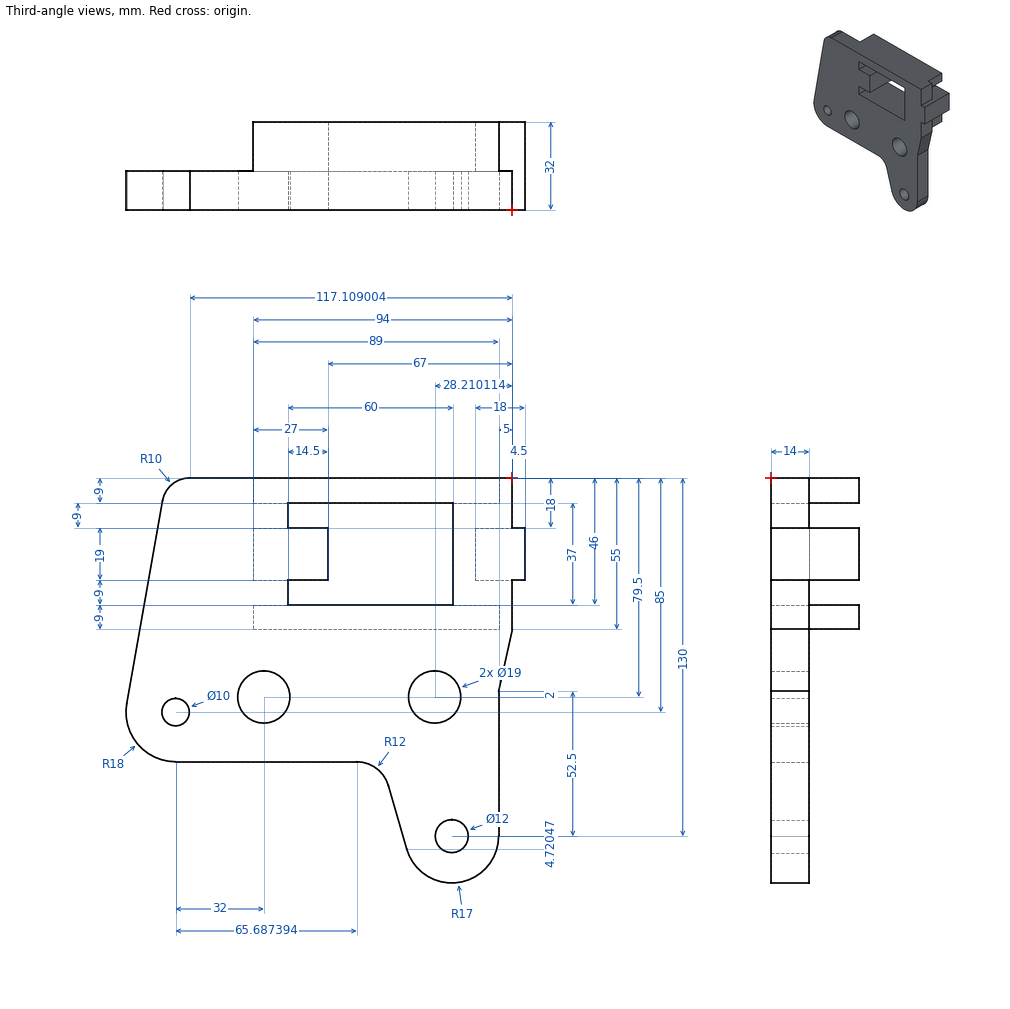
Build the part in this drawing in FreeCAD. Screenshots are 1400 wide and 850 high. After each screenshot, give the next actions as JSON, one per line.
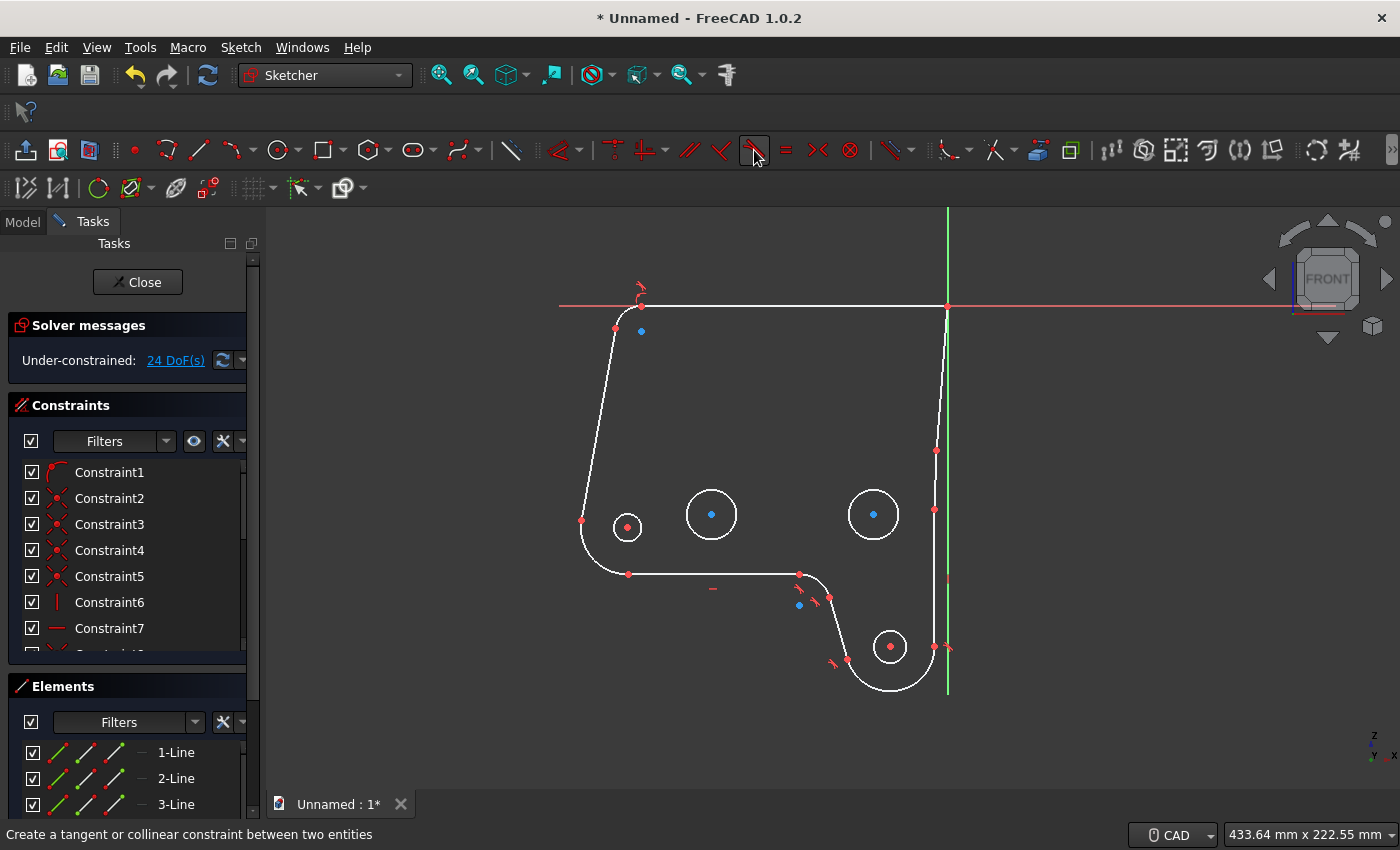
{"action": "left_click", "coordinate": [748, 574]}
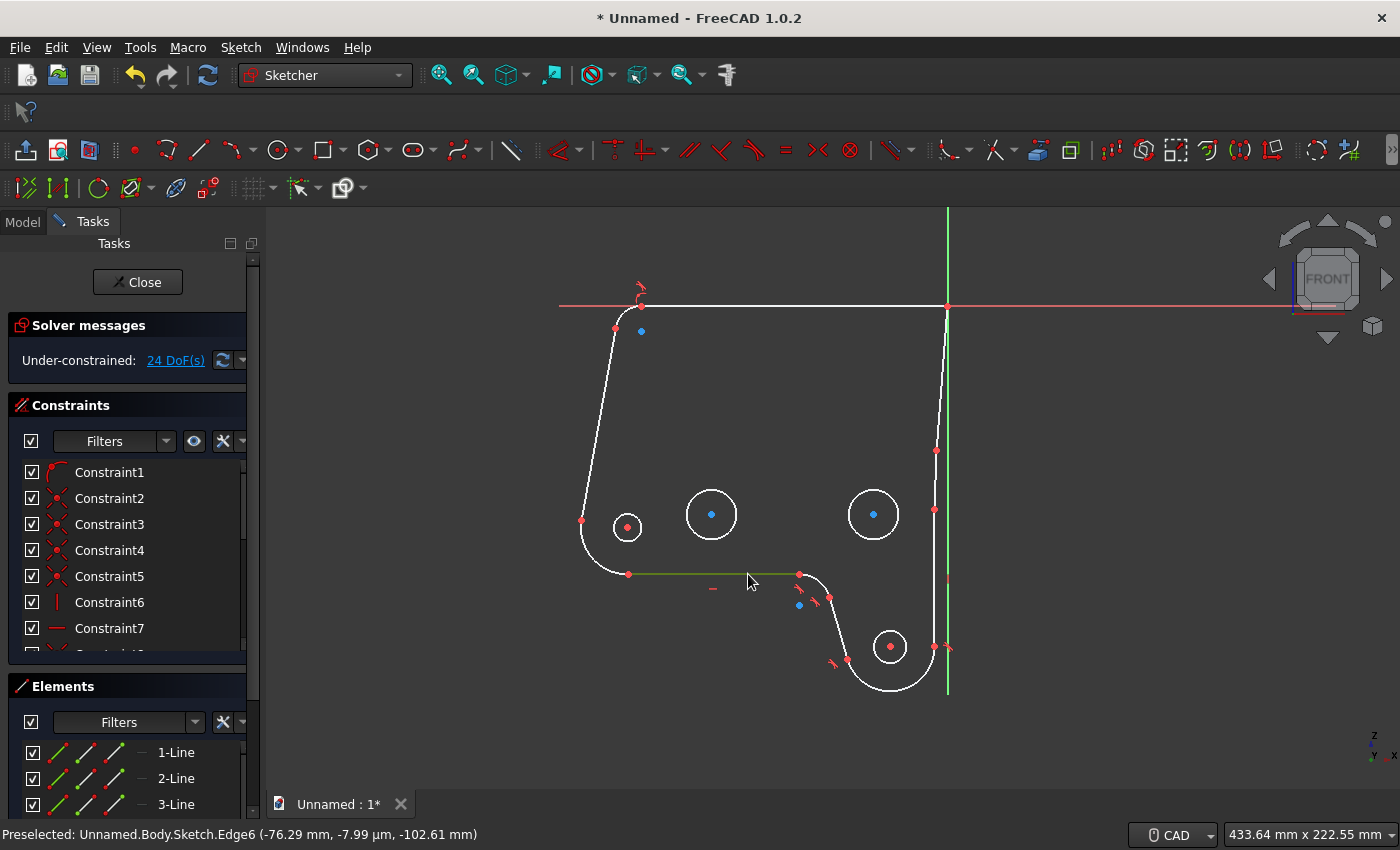
{"action": "left_click", "coordinate": [584, 545]}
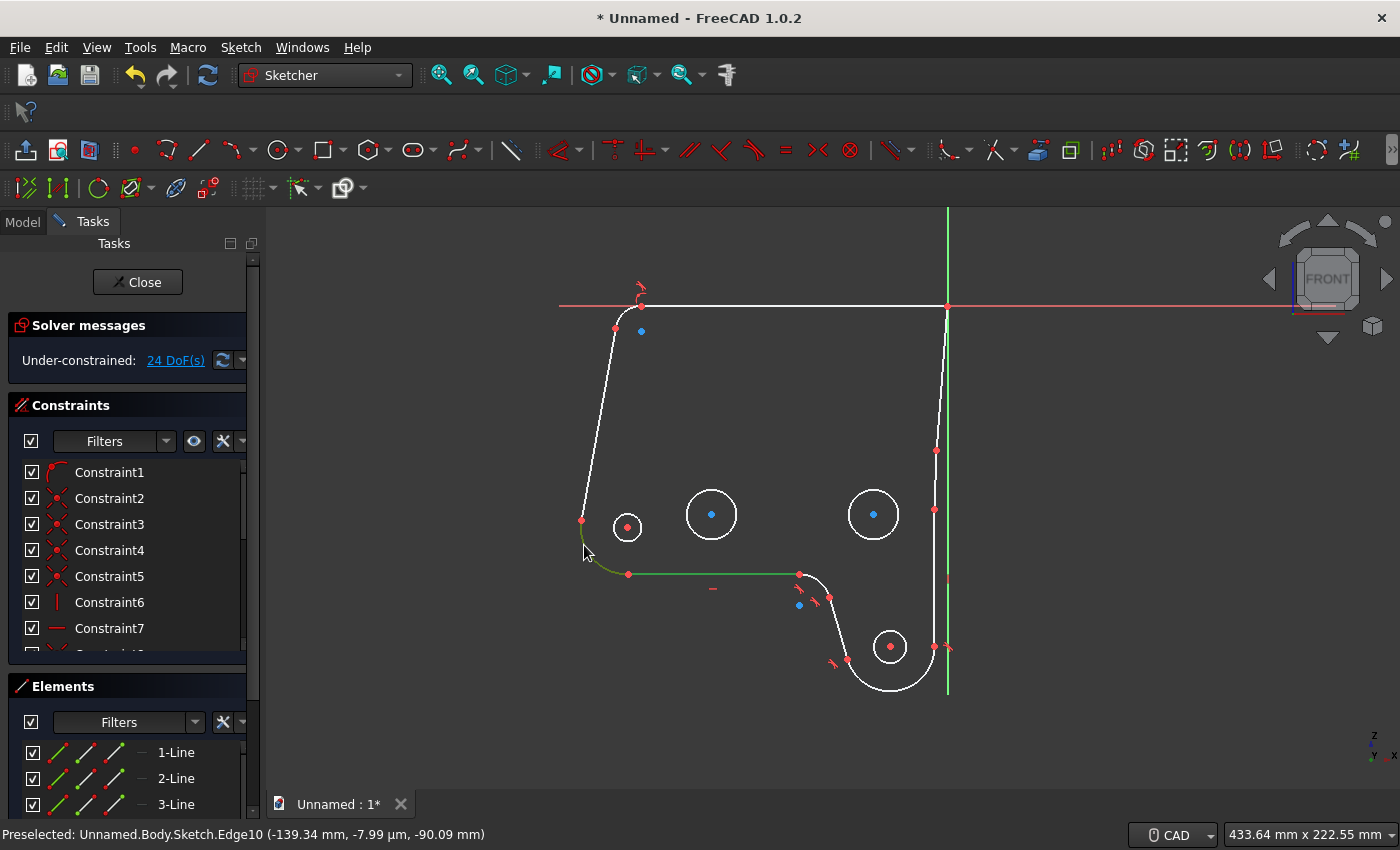
{"action": "left_click", "coordinate": [754, 150]}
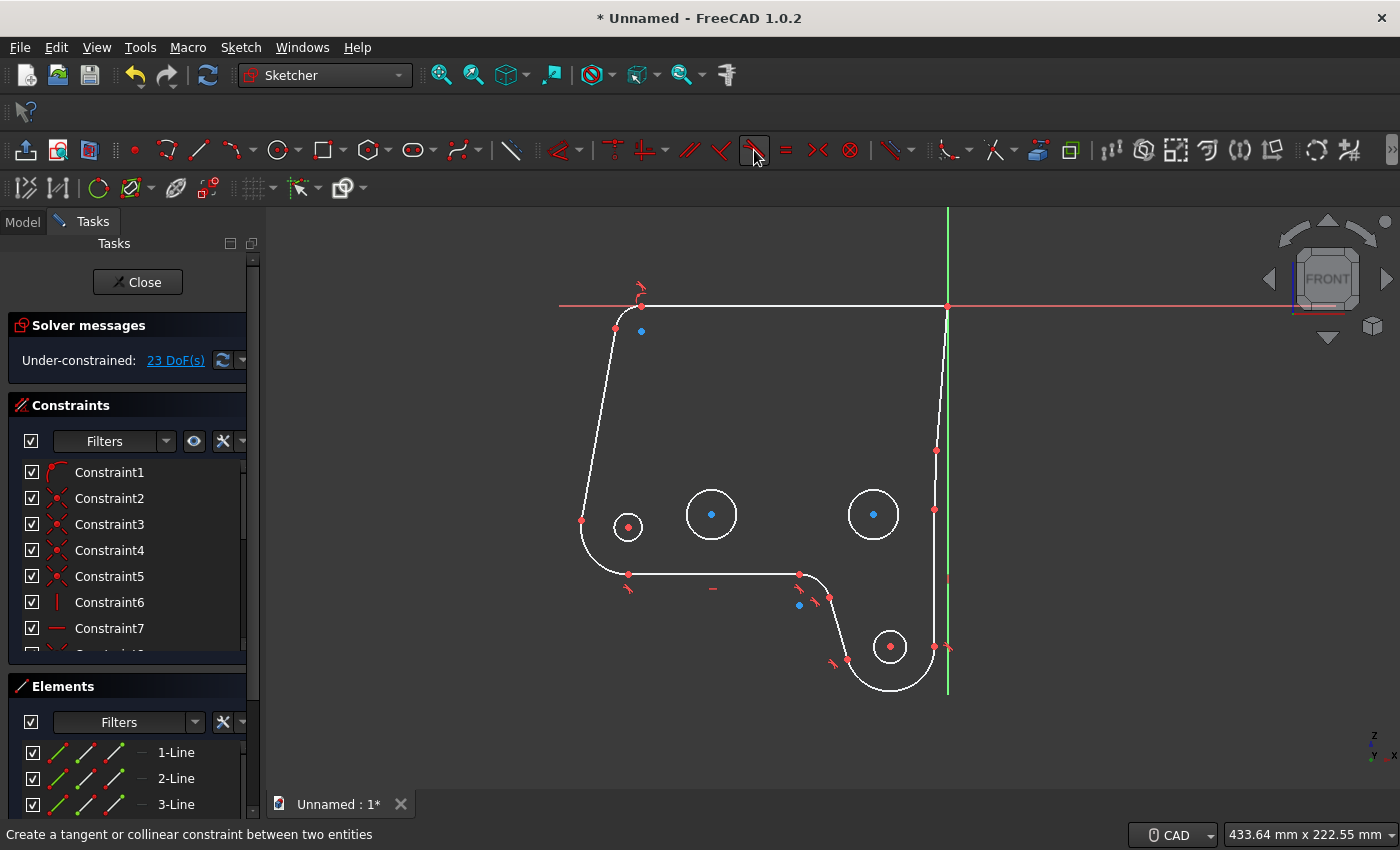
{"action": "left_click", "coordinate": [592, 463]}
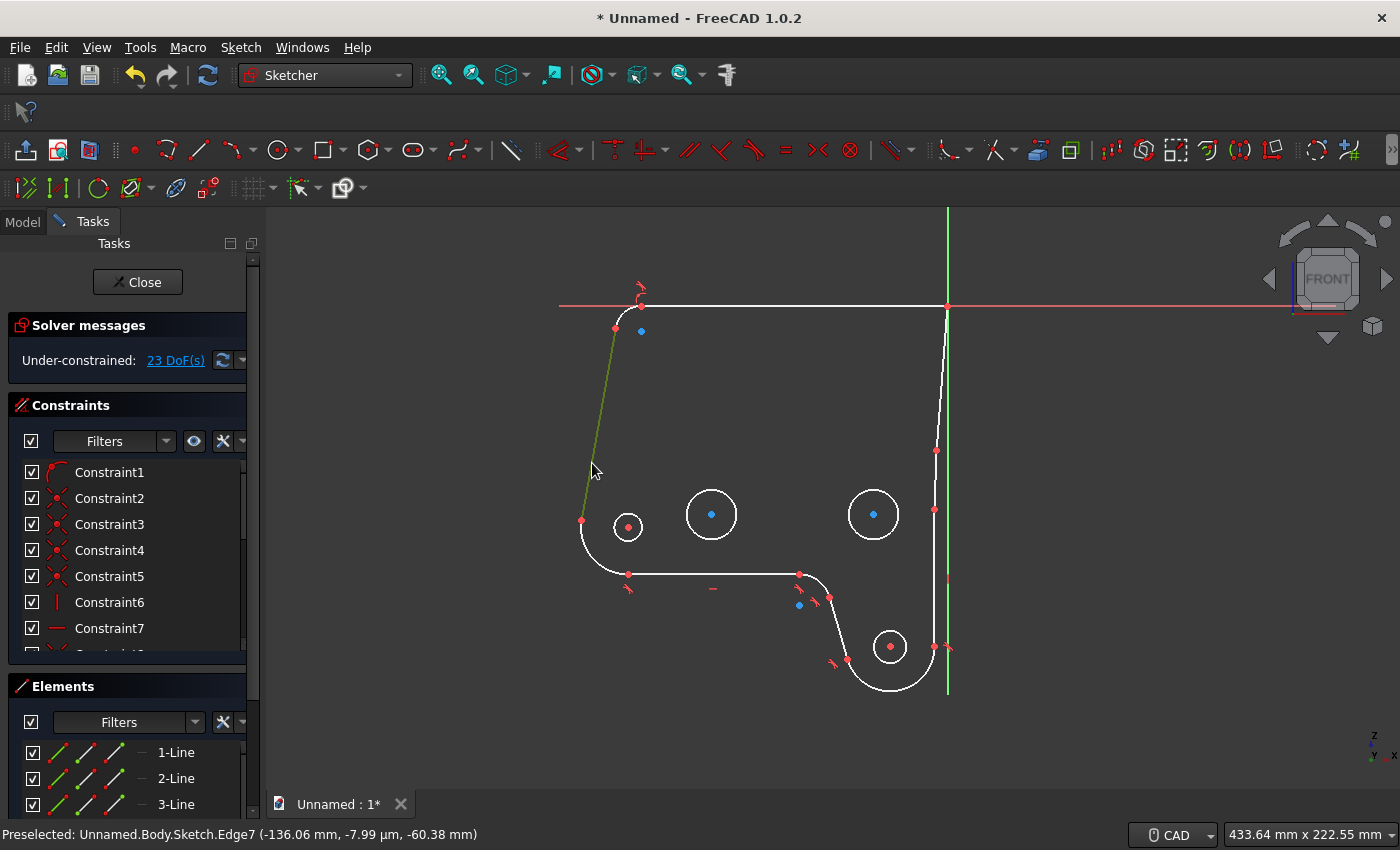
{"action": "left_click", "coordinate": [584, 545]}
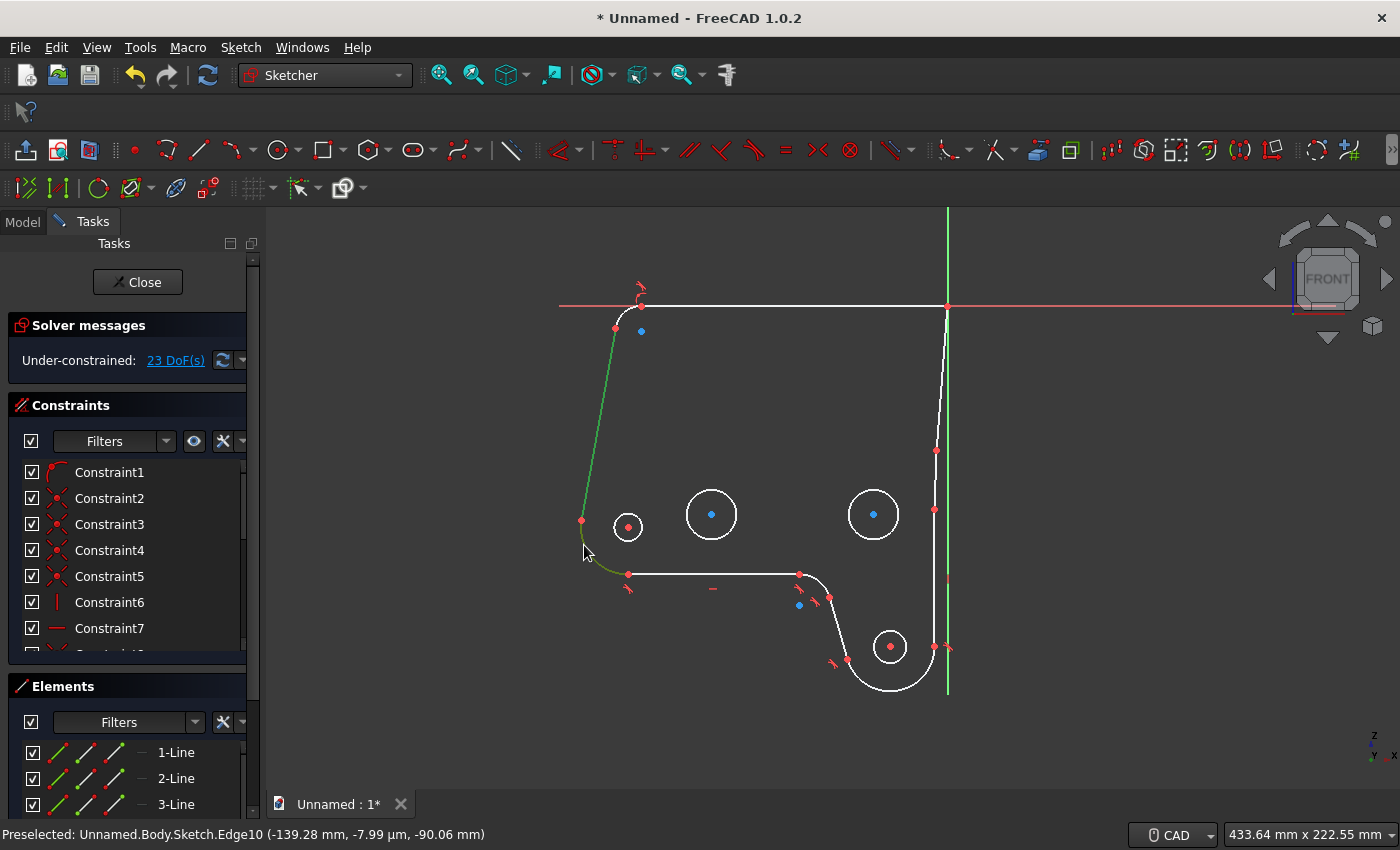
{"action": "left_click", "coordinate": [754, 150]}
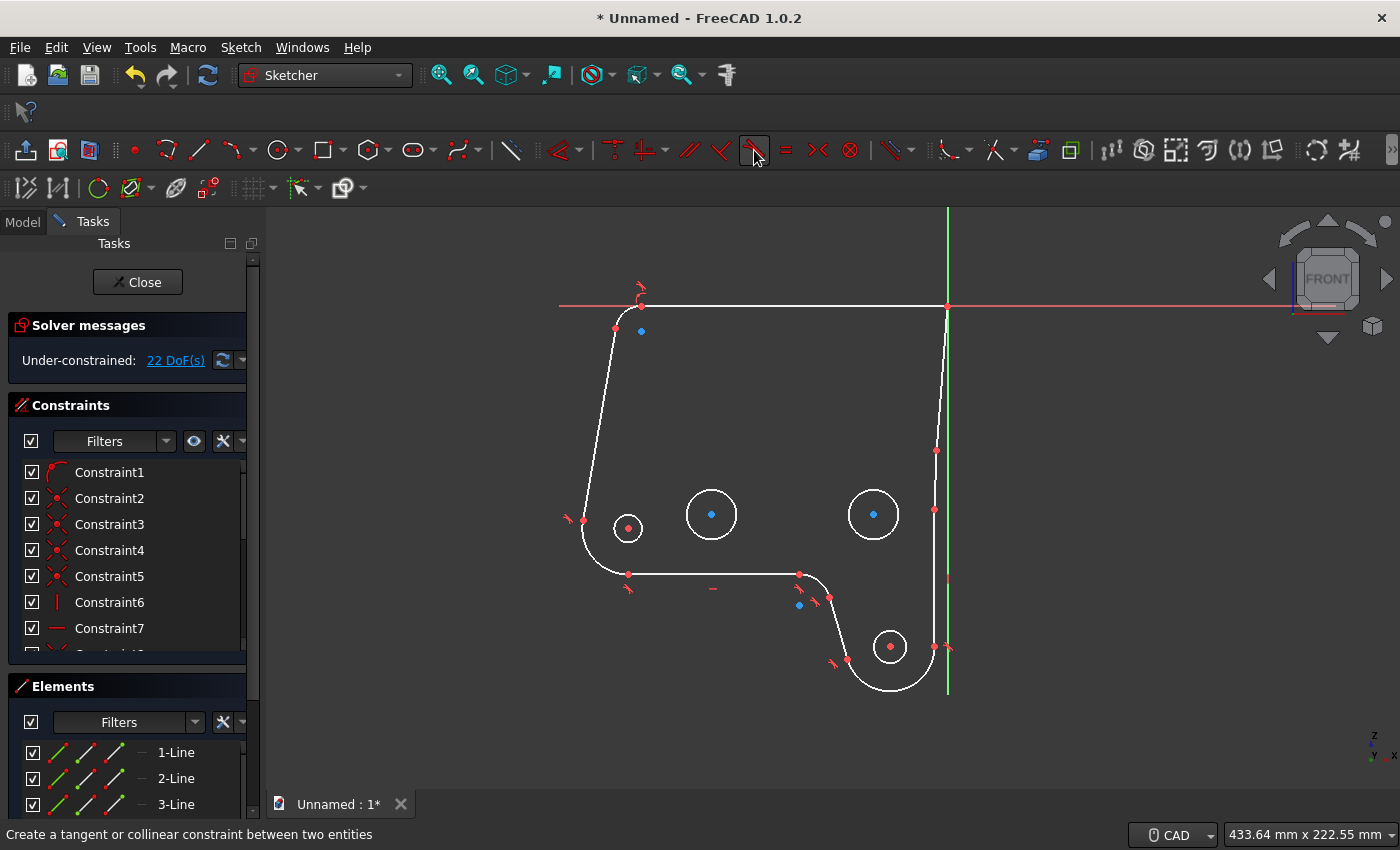
{"action": "left_click", "coordinate": [593, 463]}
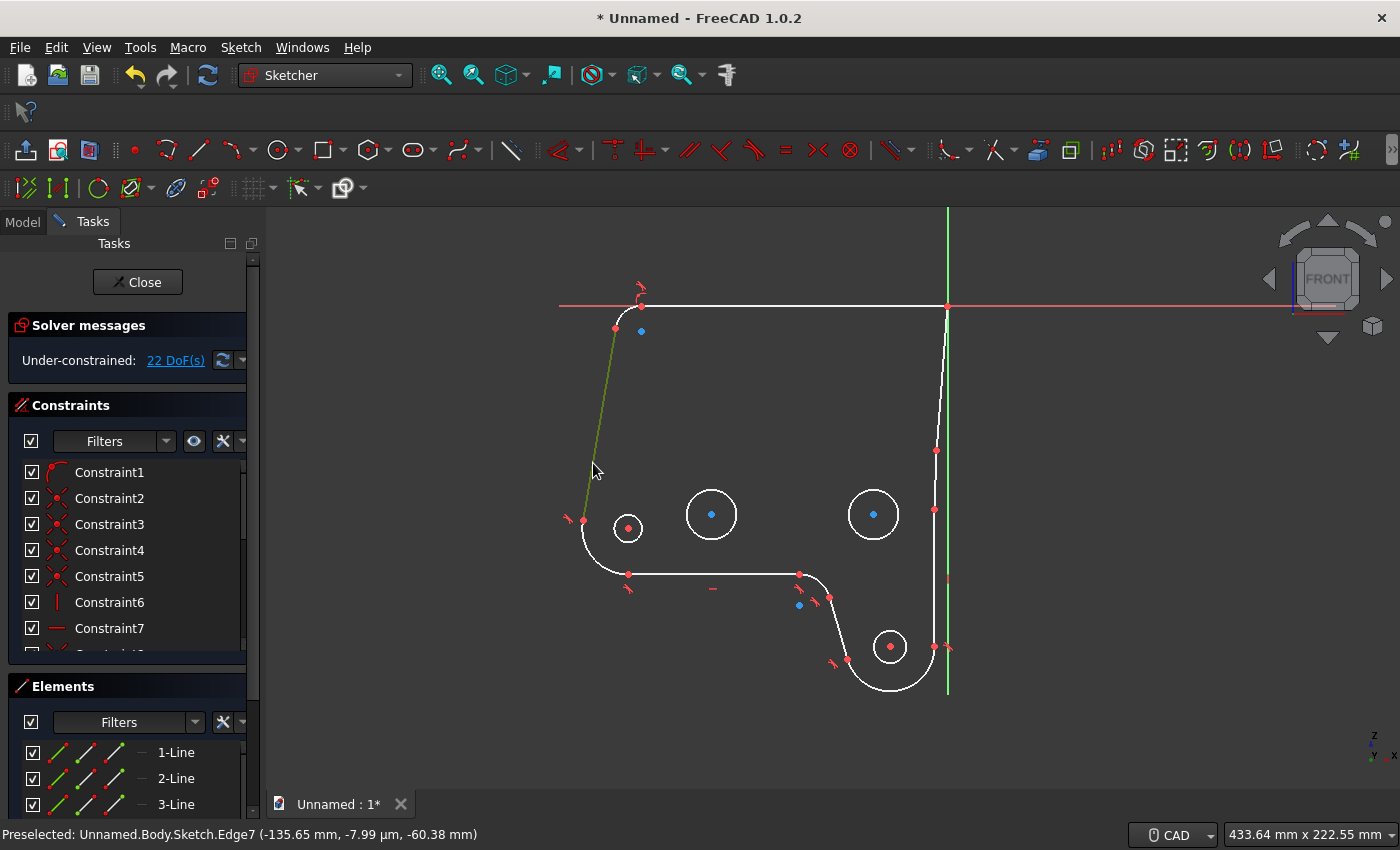
{"action": "scroll", "coordinate": [630, 308], "scroll_direction": "up", "scroll_amount": 2}